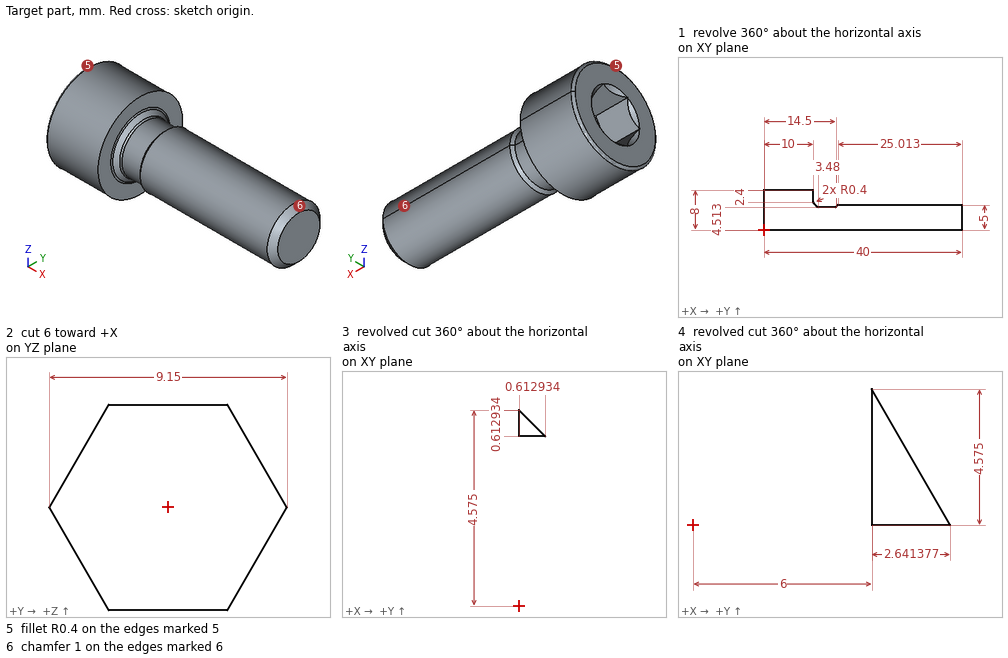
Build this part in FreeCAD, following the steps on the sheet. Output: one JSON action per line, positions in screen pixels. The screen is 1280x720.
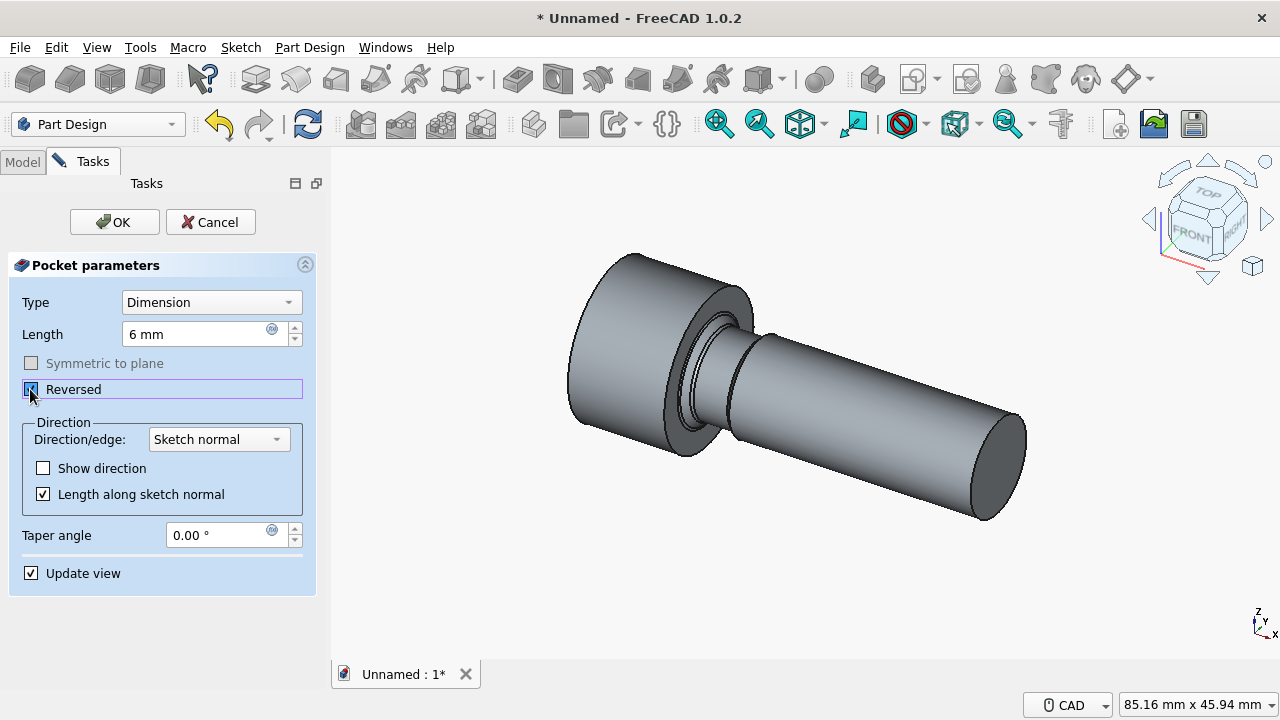
{"action": "left_click", "coordinate": [115, 222]}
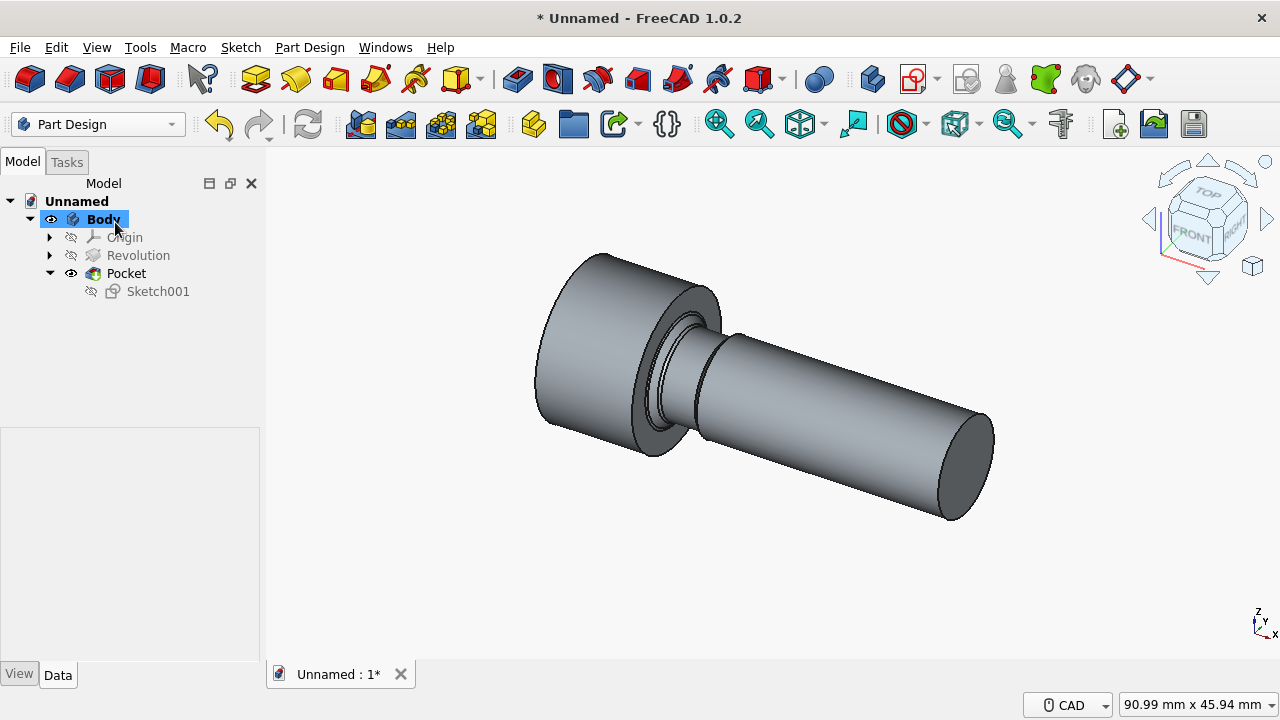
{"action": "left_click", "coordinate": [914, 80]}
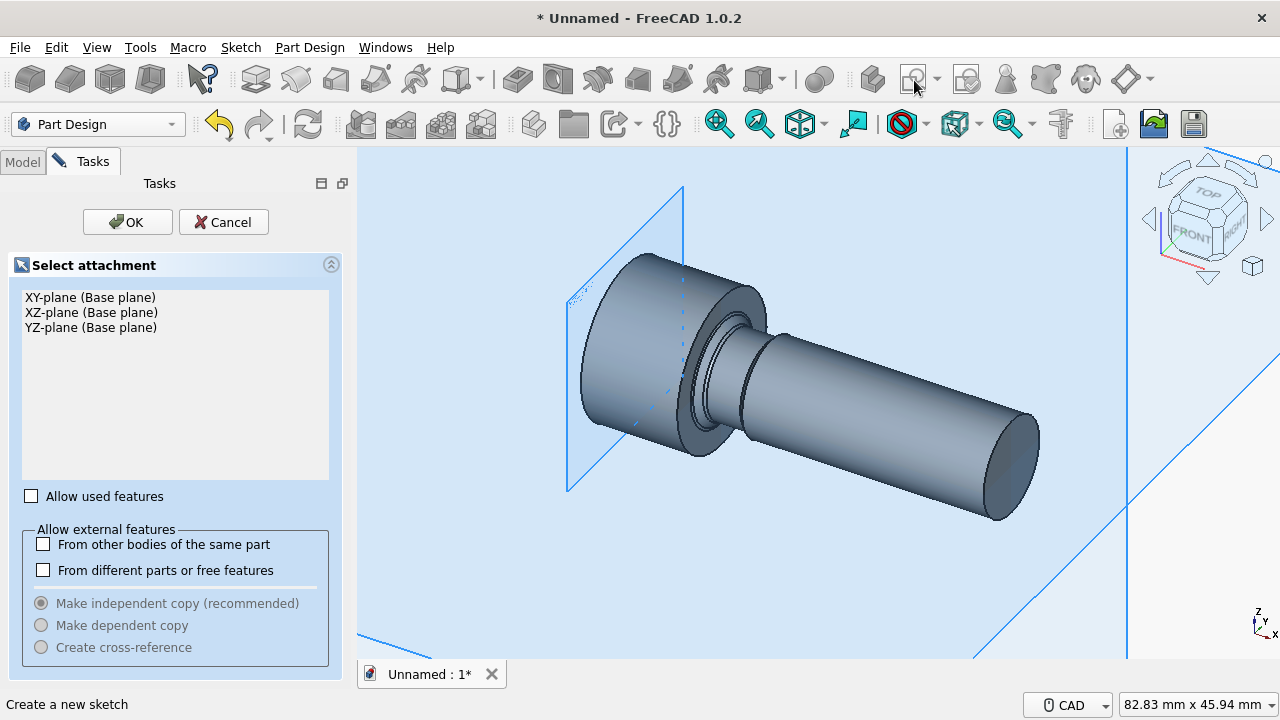
{"action": "left_click", "coordinate": [82, 298]}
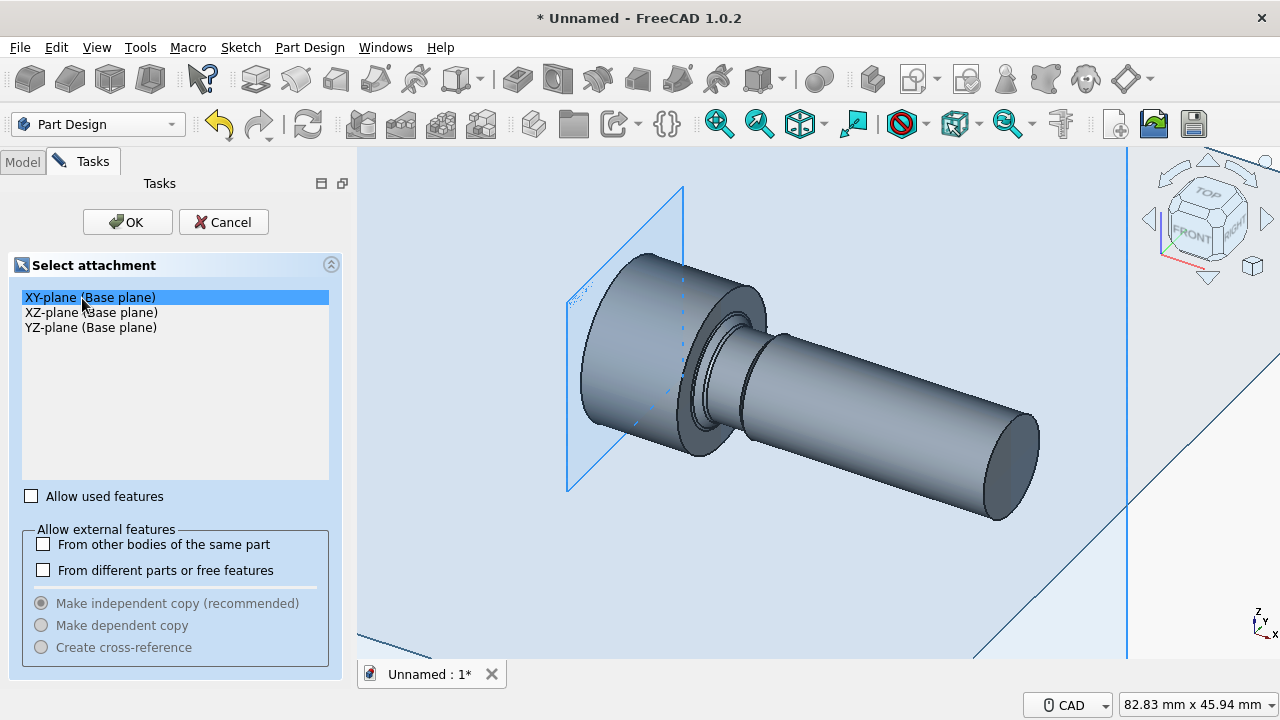
{"action": "left_click", "coordinate": [128, 222]}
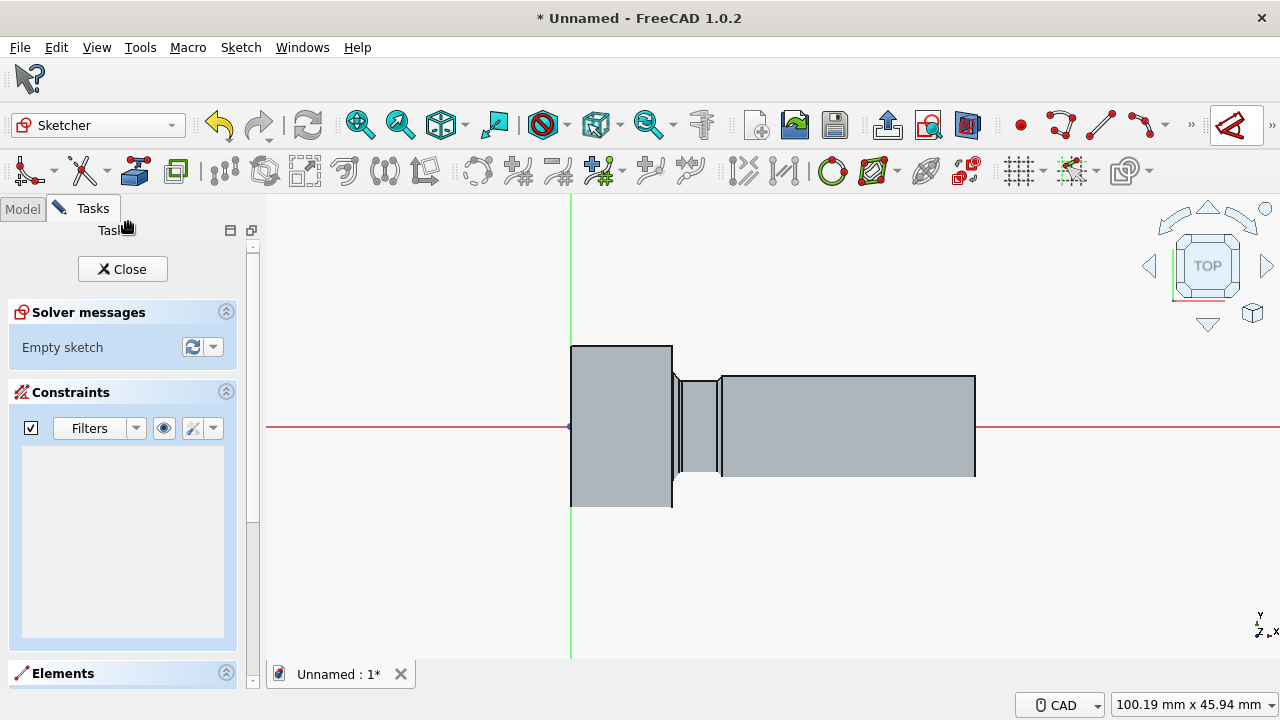
{"action": "left_click", "coordinate": [968, 126]}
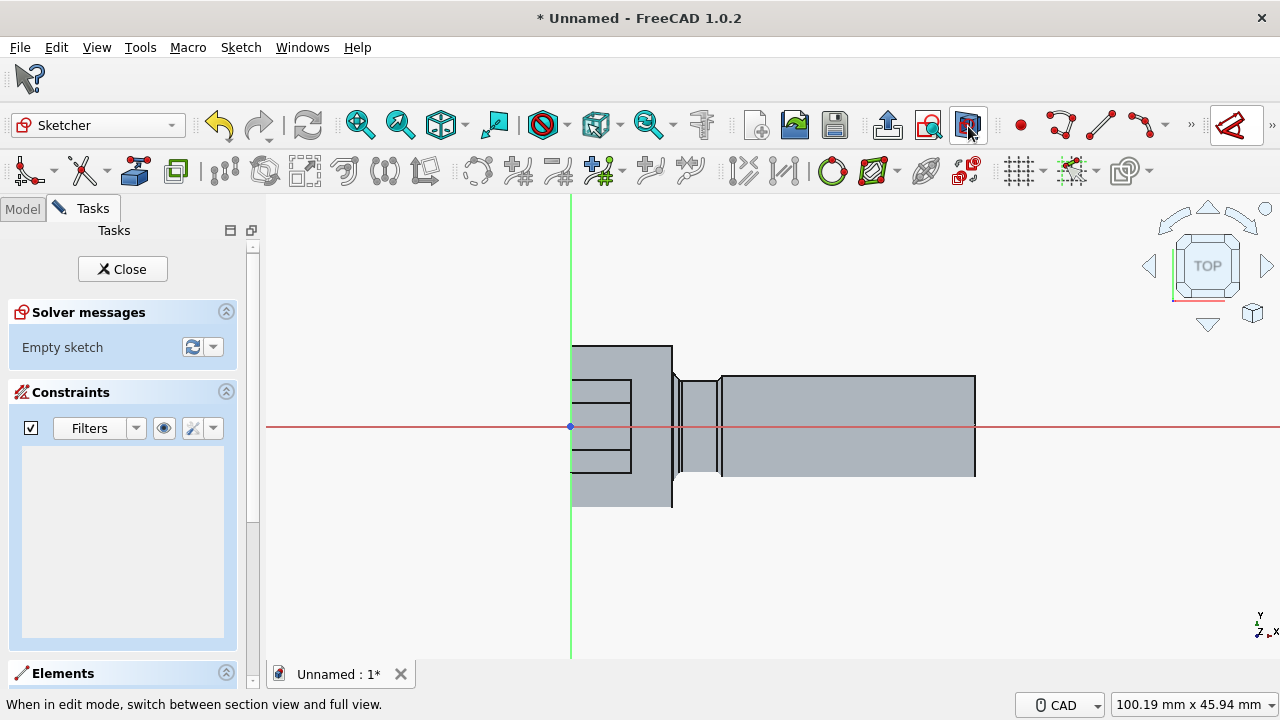
{"action": "scroll", "coordinate": [567, 381], "scroll_direction": "up", "scroll_amount": 15}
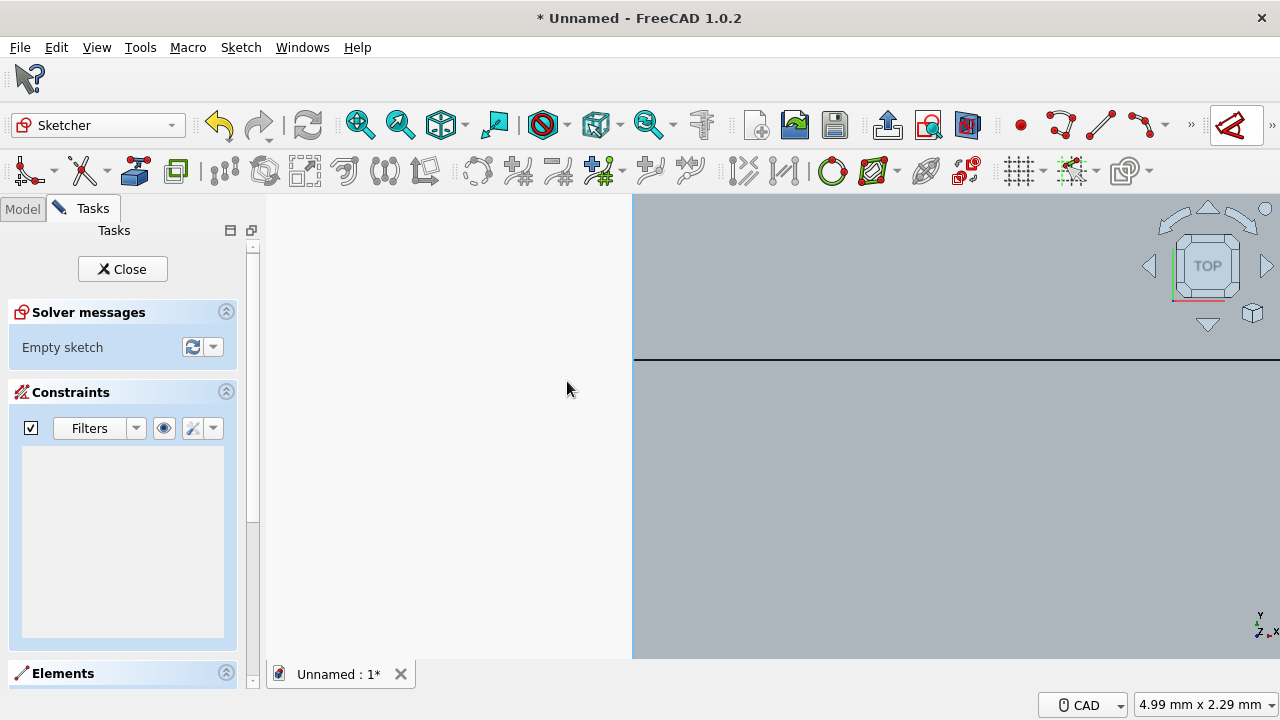
{"action": "scroll", "coordinate": [688, 418], "scroll_direction": "up", "scroll_amount": 4}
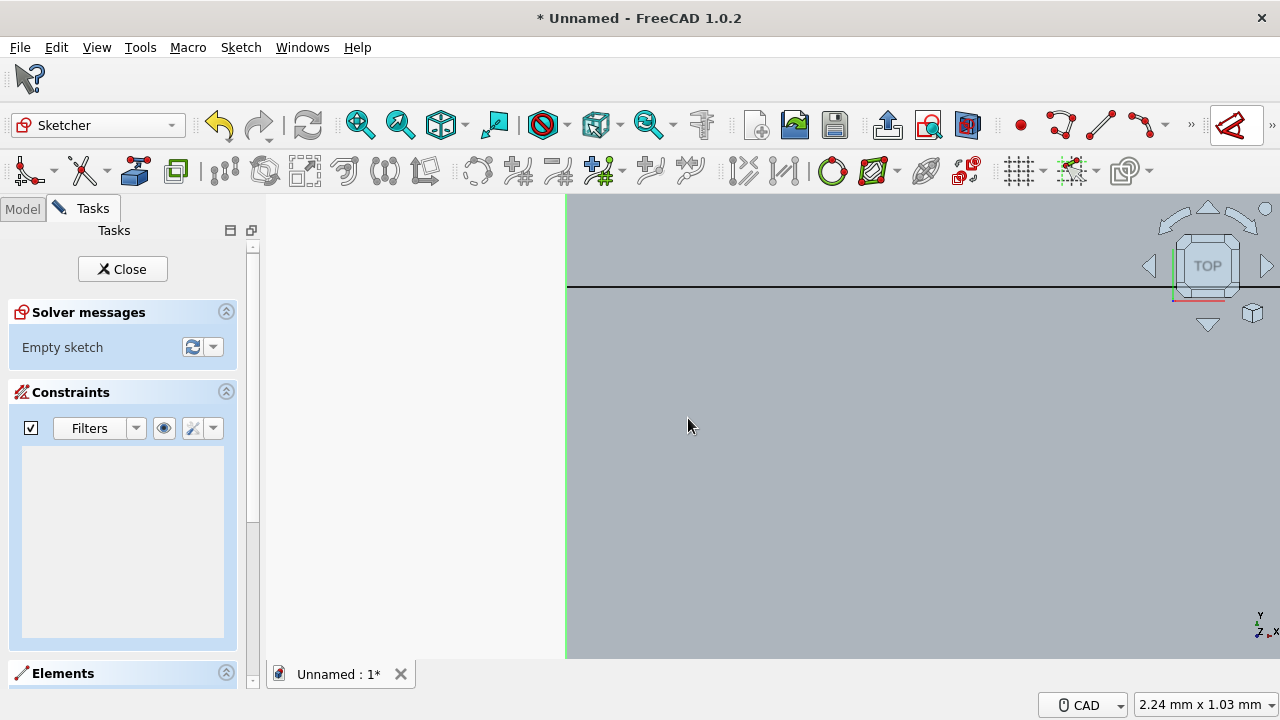
{"action": "left_click", "coordinate": [1062, 126]}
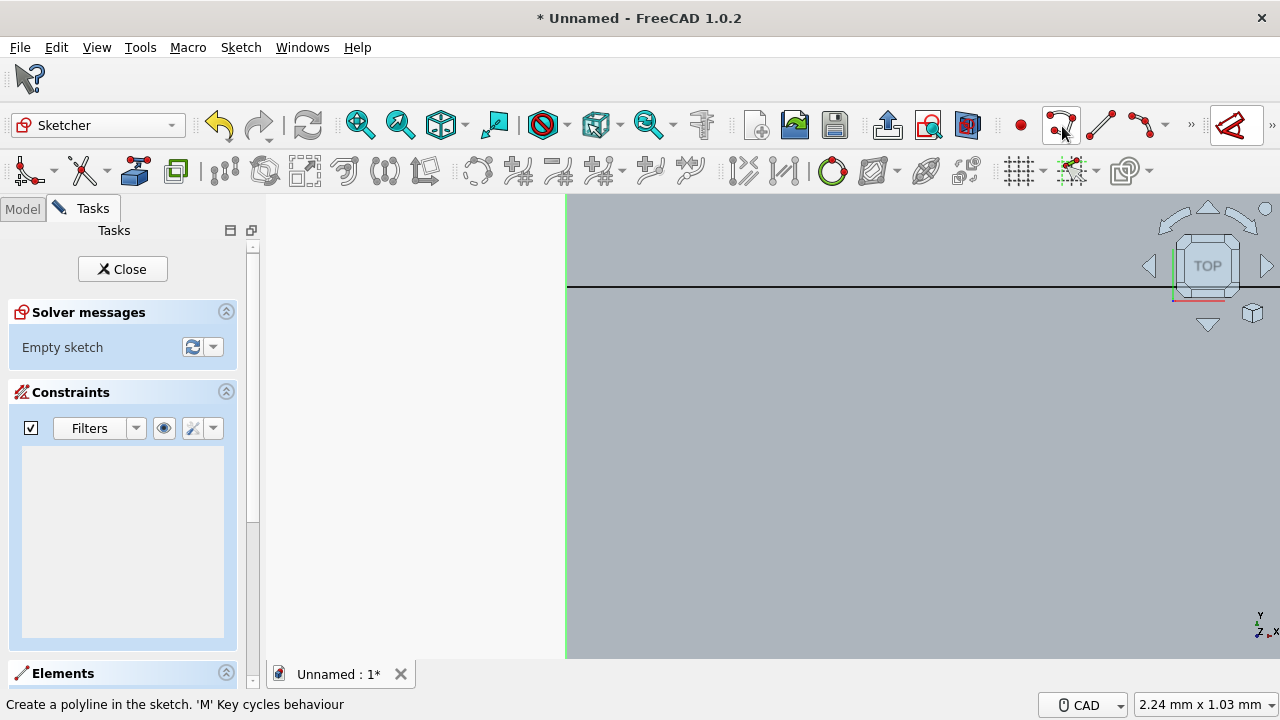
{"action": "left_click", "coordinate": [566, 565]}
{"action": "left_click", "coordinate": [843, 565]}
{"action": "left_click", "coordinate": [575, 287]}
{"action": "left_click", "coordinate": [566, 566]}
{"action": "key", "text": "Escape"}
{"action": "key", "text": "Escape"}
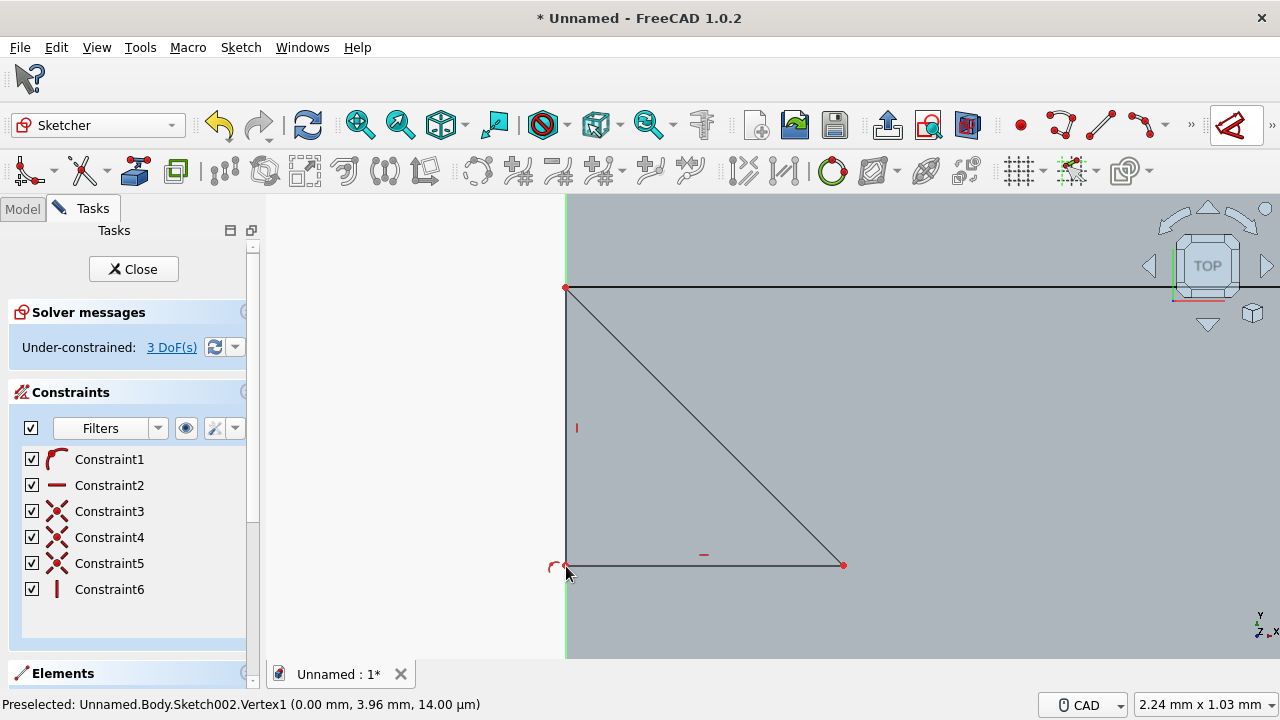
{"action": "left_click", "coordinate": [566, 288]}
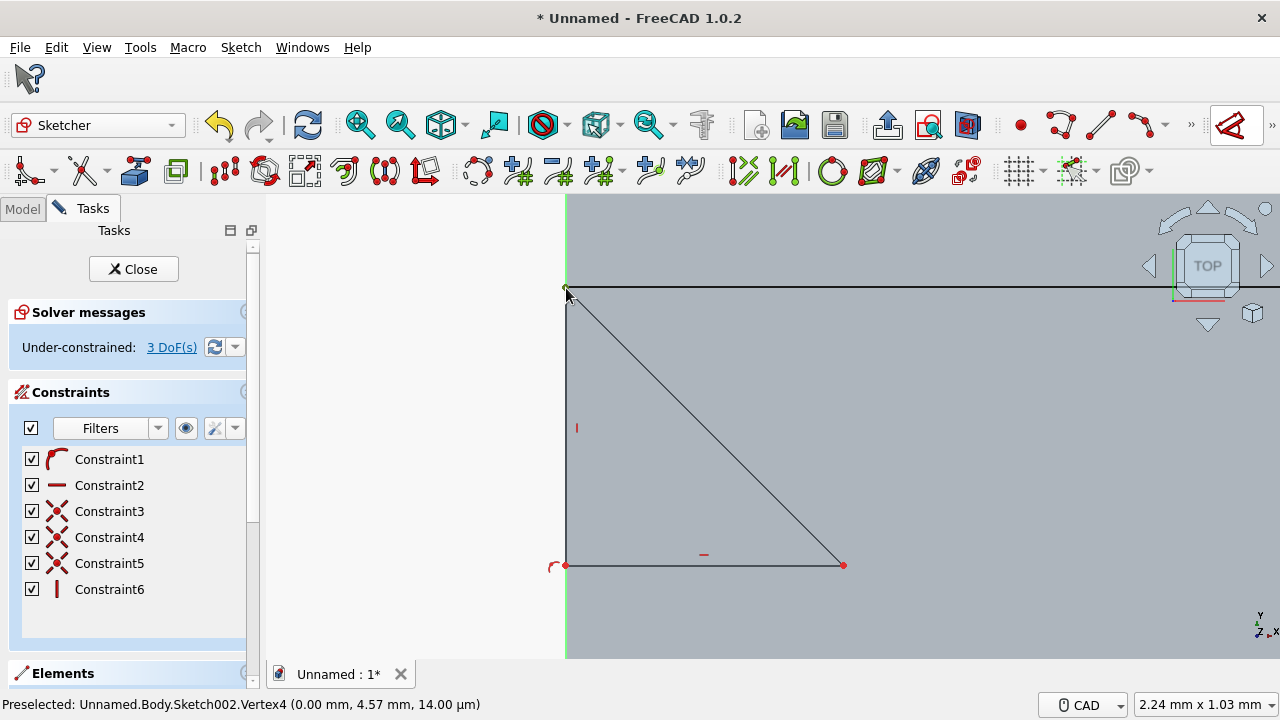
{"action": "left_click", "coordinate": [1258, 126]}